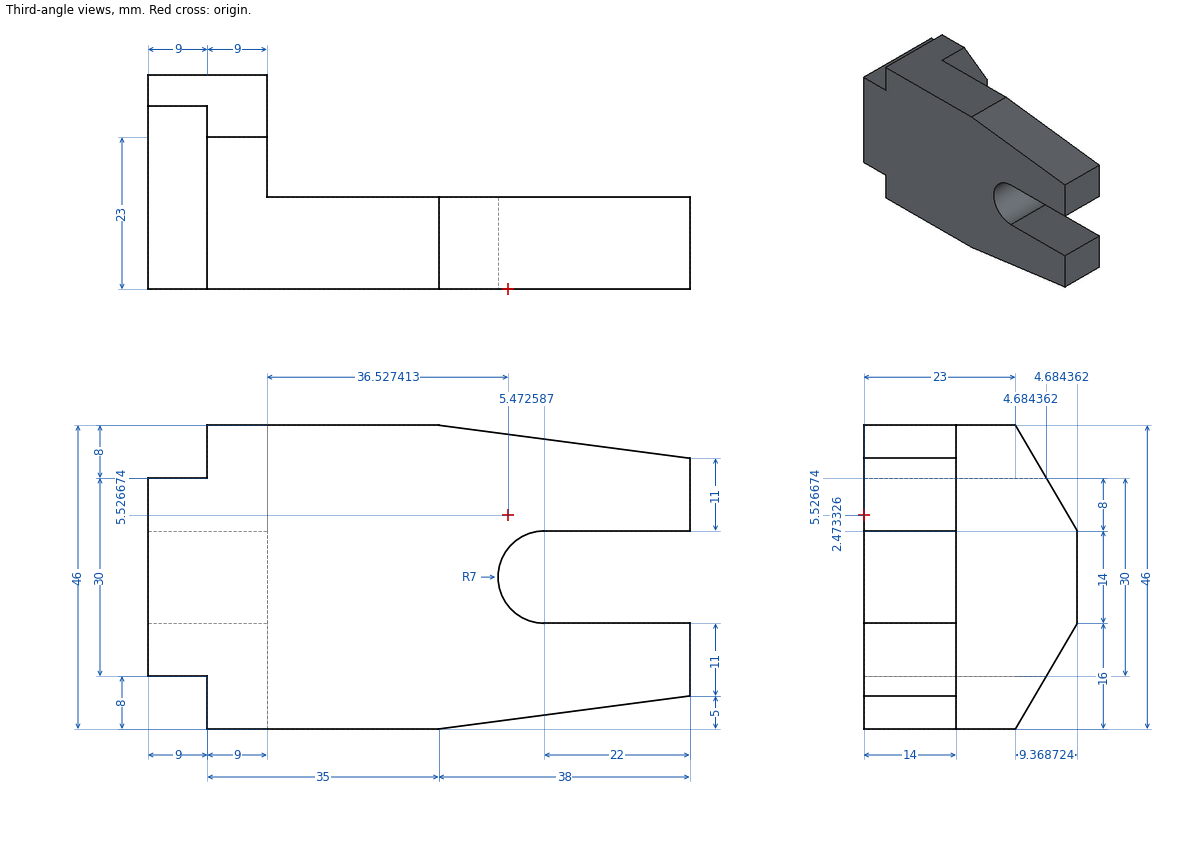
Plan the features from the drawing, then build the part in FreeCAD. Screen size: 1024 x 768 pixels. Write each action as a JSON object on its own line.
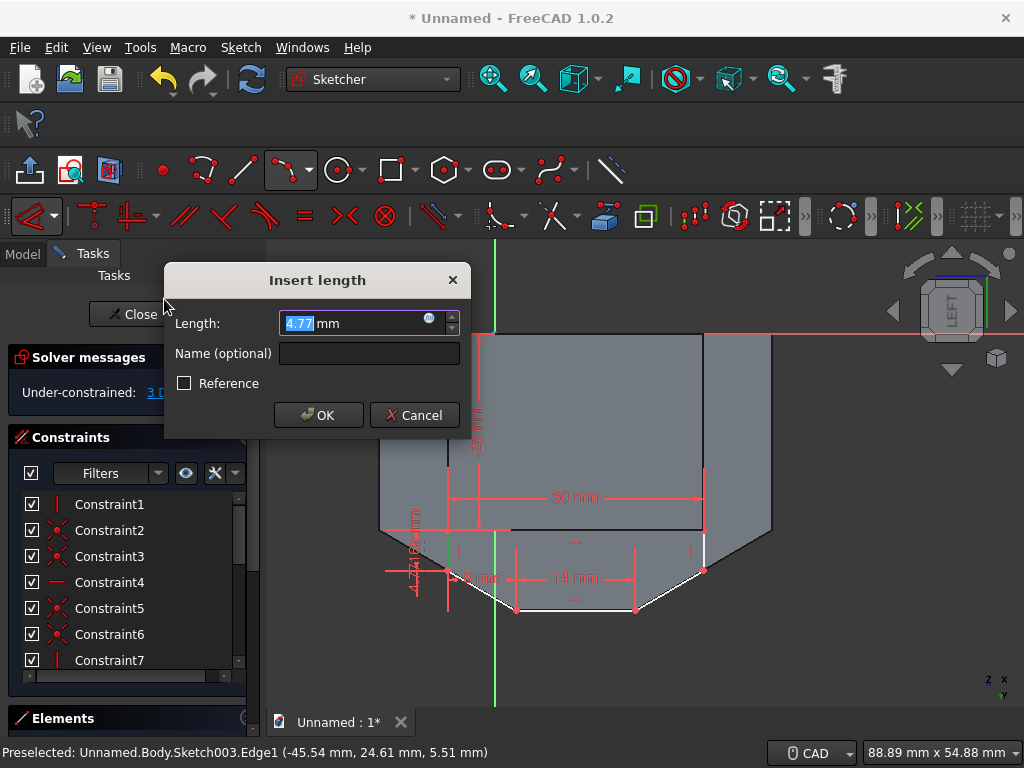
{"action": "type", "text": "4.684362"}
{"action": "key", "text": "Return"}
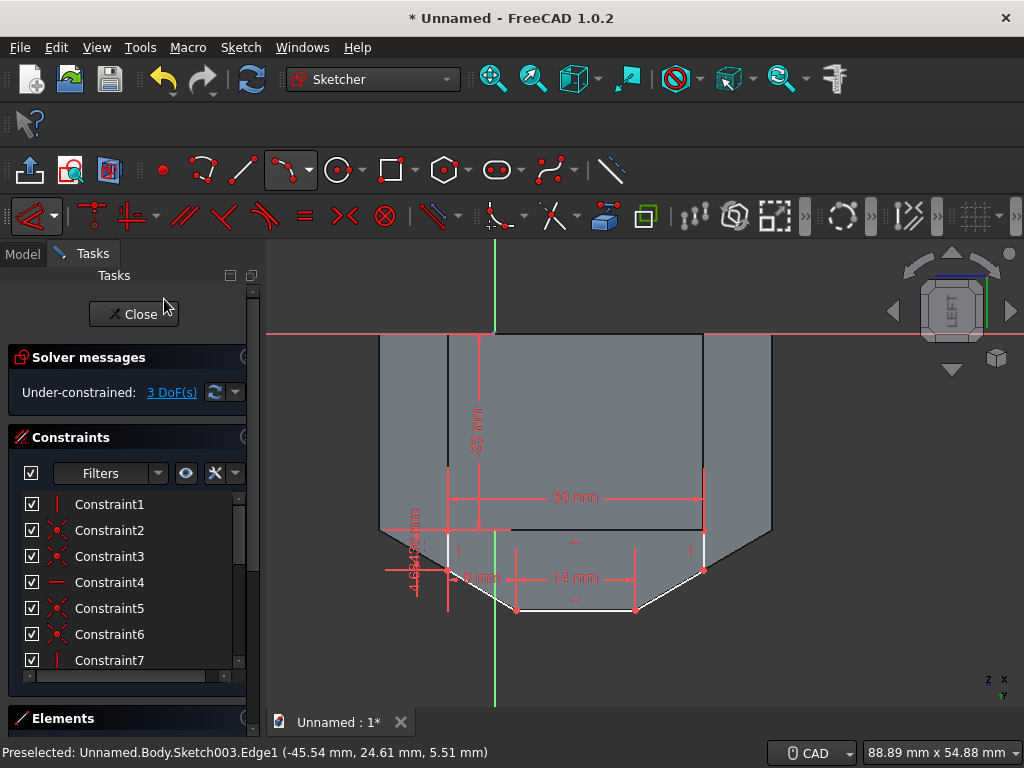
{"action": "left_click", "coordinate": [704, 559]}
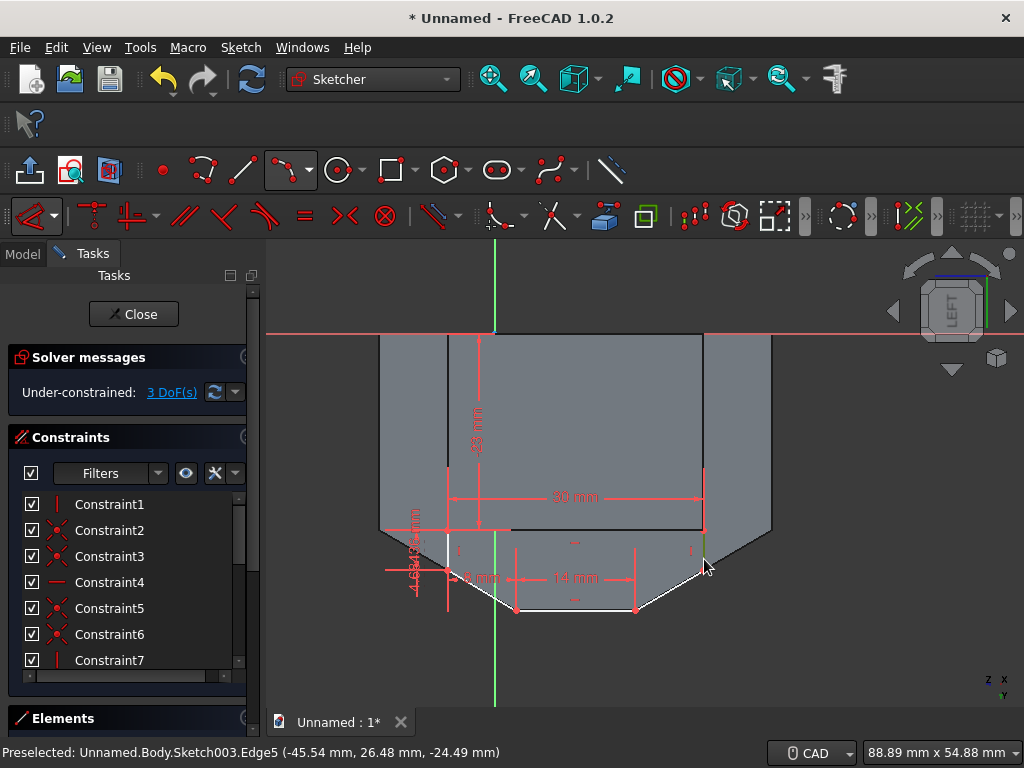
{"action": "left_click", "coordinate": [56, 216]}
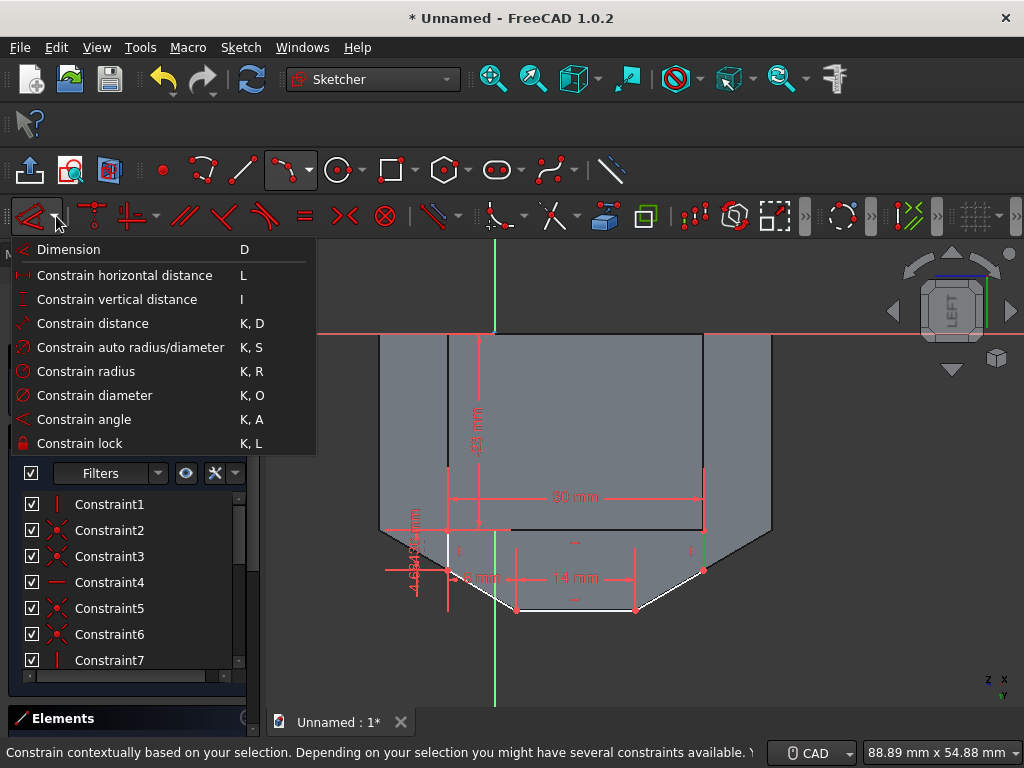
{"action": "left_click", "coordinate": [164, 299]}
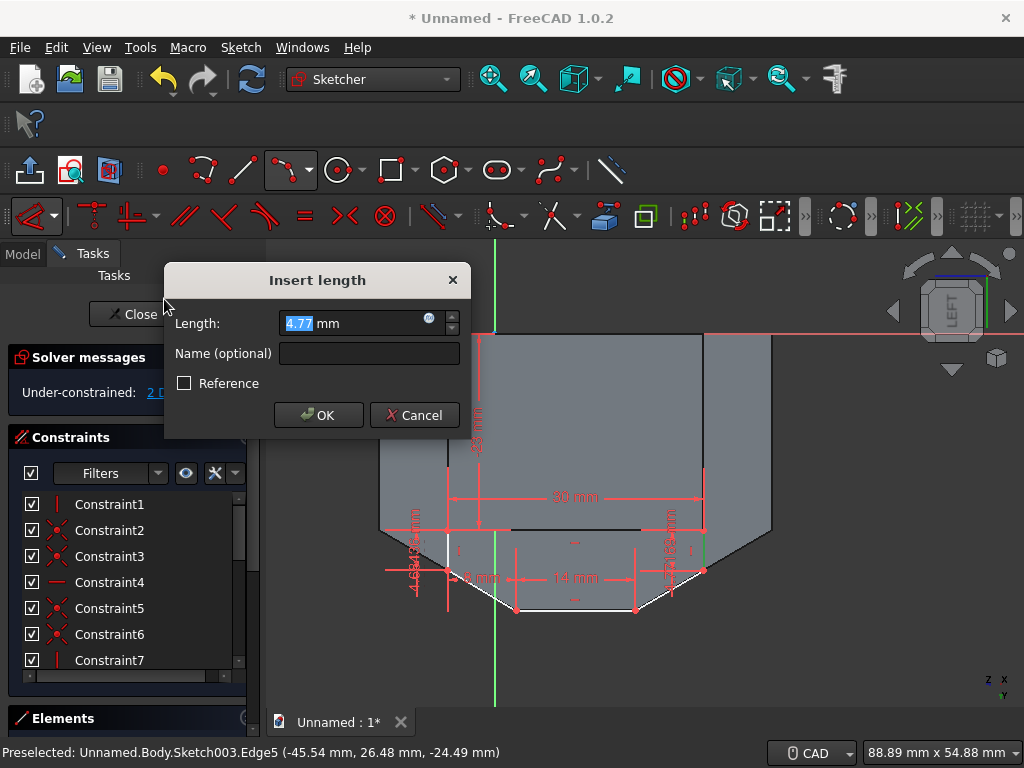
{"action": "type", "text": "4.684362"}
{"action": "key", "text": "Return"}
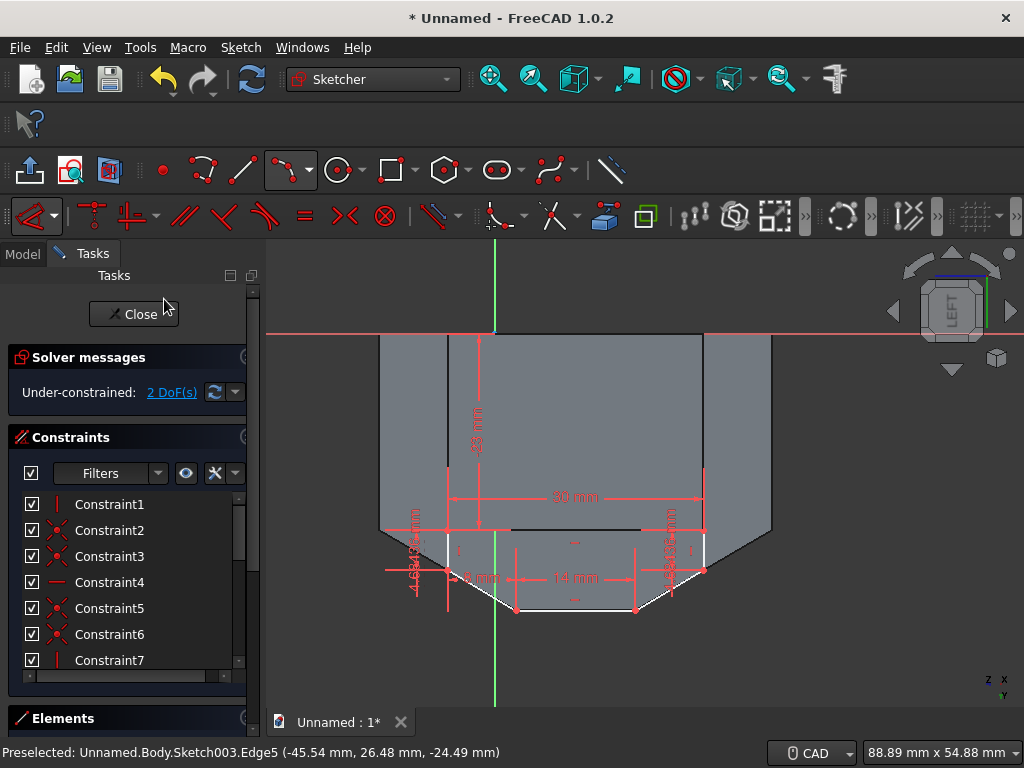
{"action": "left_click", "coordinate": [448, 530]}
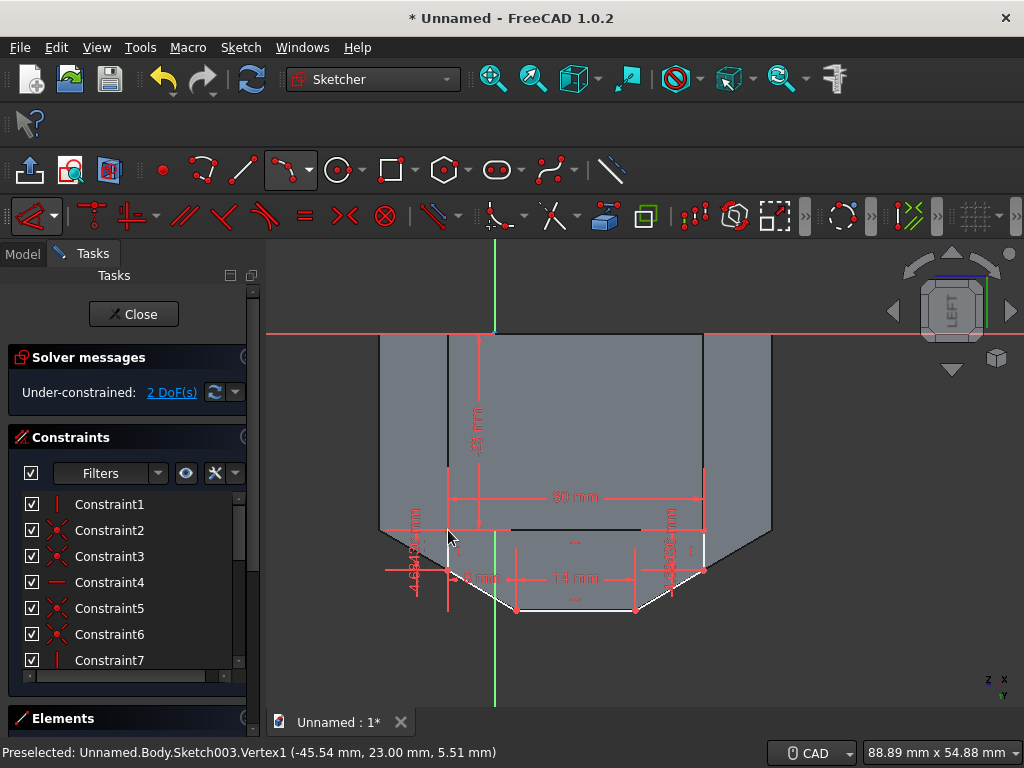
{"action": "left_click", "coordinate": [56, 216]}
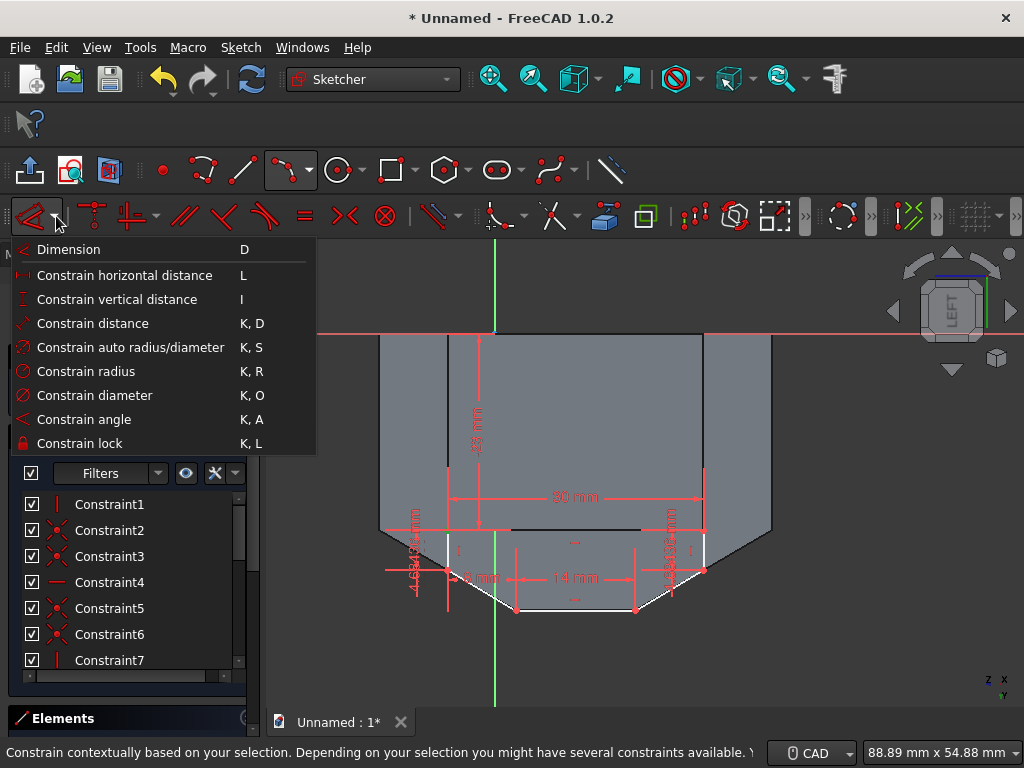
{"action": "left_click", "coordinate": [164, 275]}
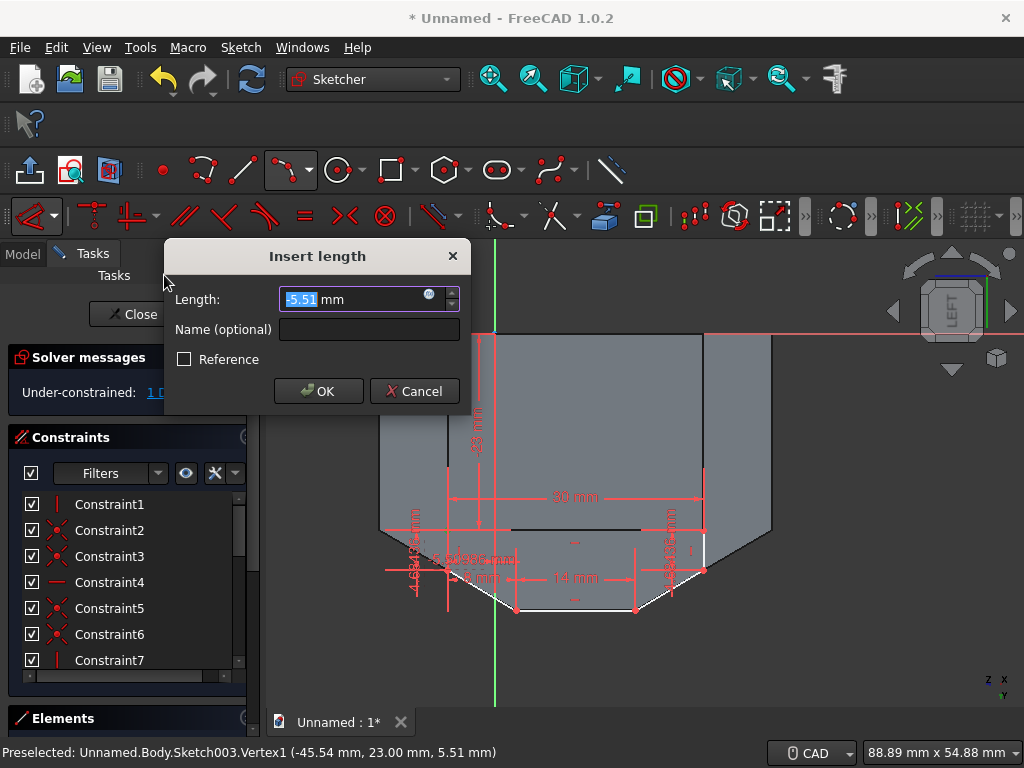
{"action": "type", "text": "-5.526674"}
{"action": "key", "text": "Return"}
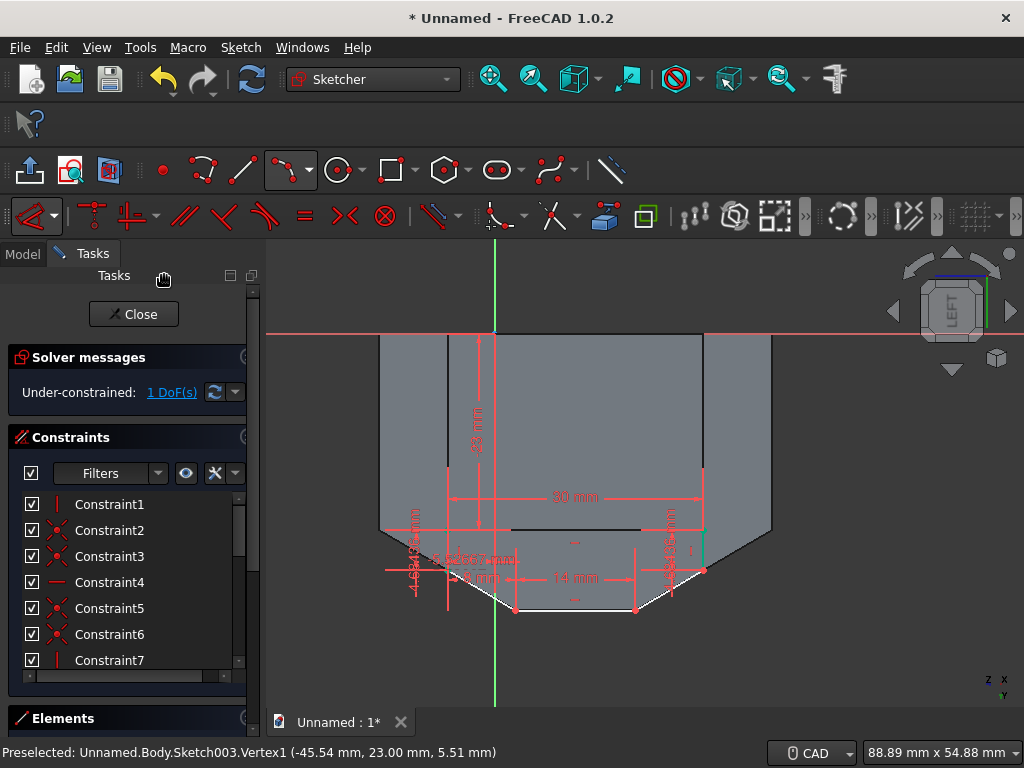
{"action": "left_click", "coordinate": [495, 599]}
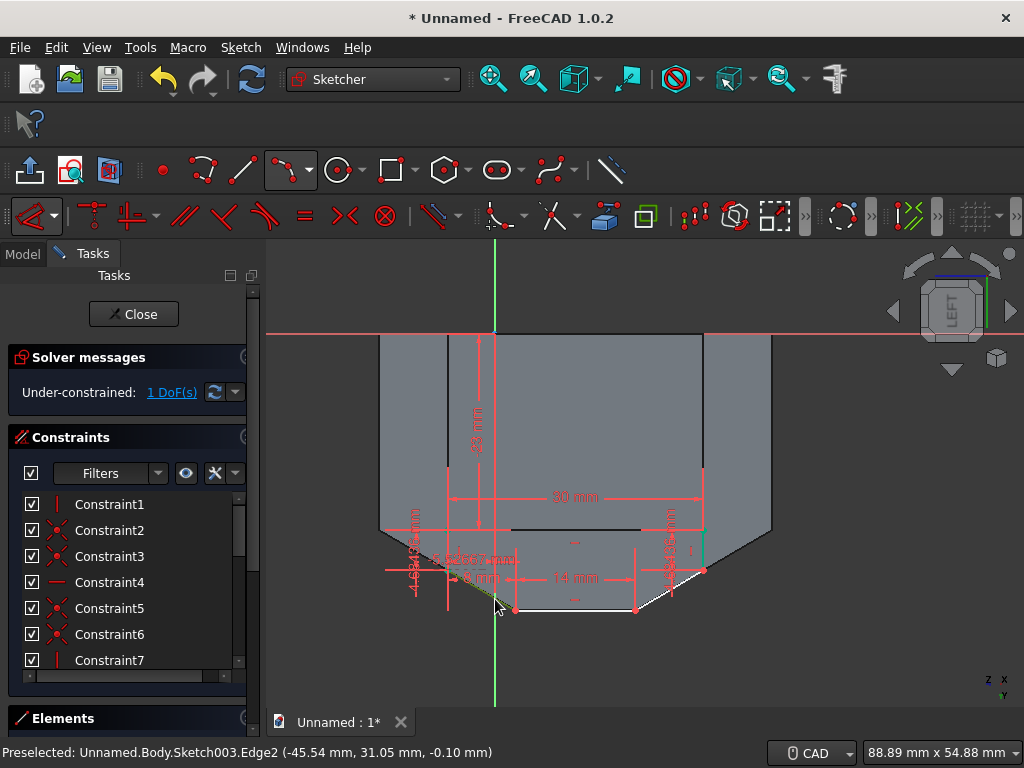
{"action": "left_click", "coordinate": [56, 216]}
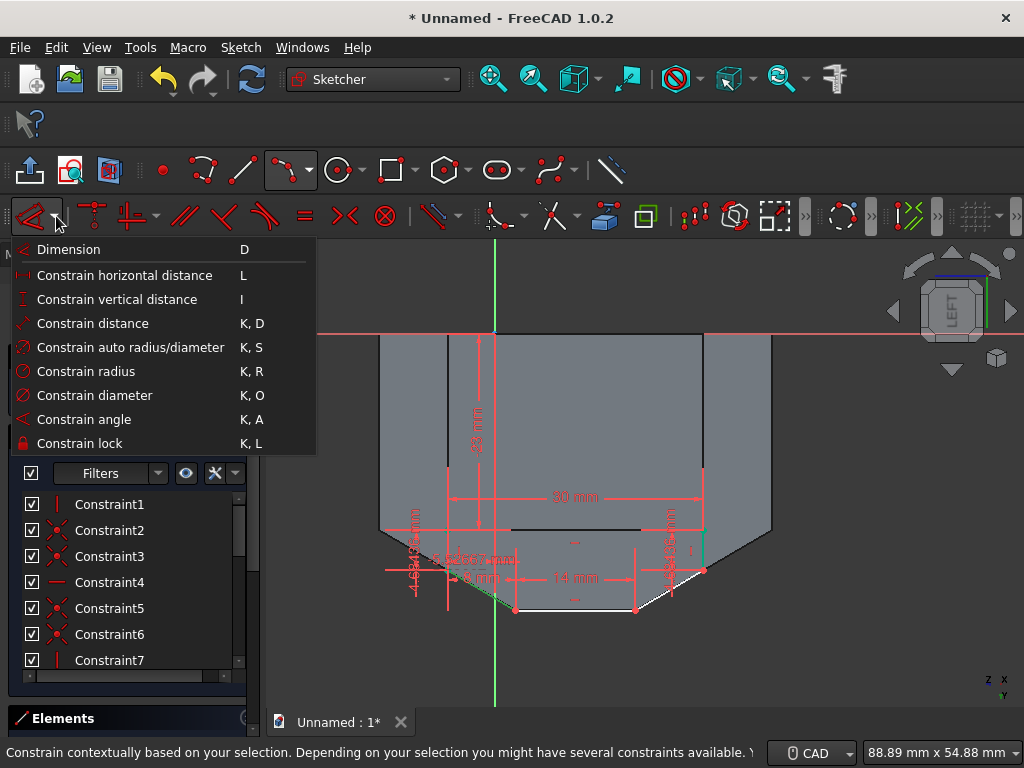
{"action": "left_click", "coordinate": [164, 299]}